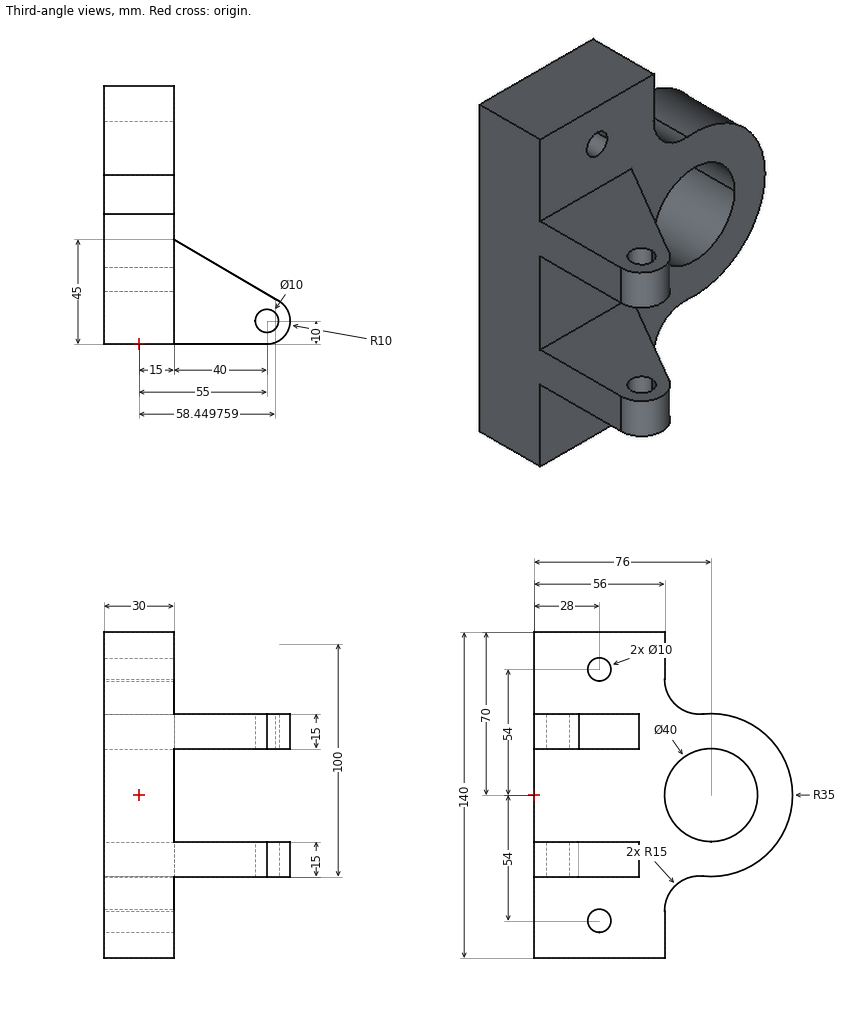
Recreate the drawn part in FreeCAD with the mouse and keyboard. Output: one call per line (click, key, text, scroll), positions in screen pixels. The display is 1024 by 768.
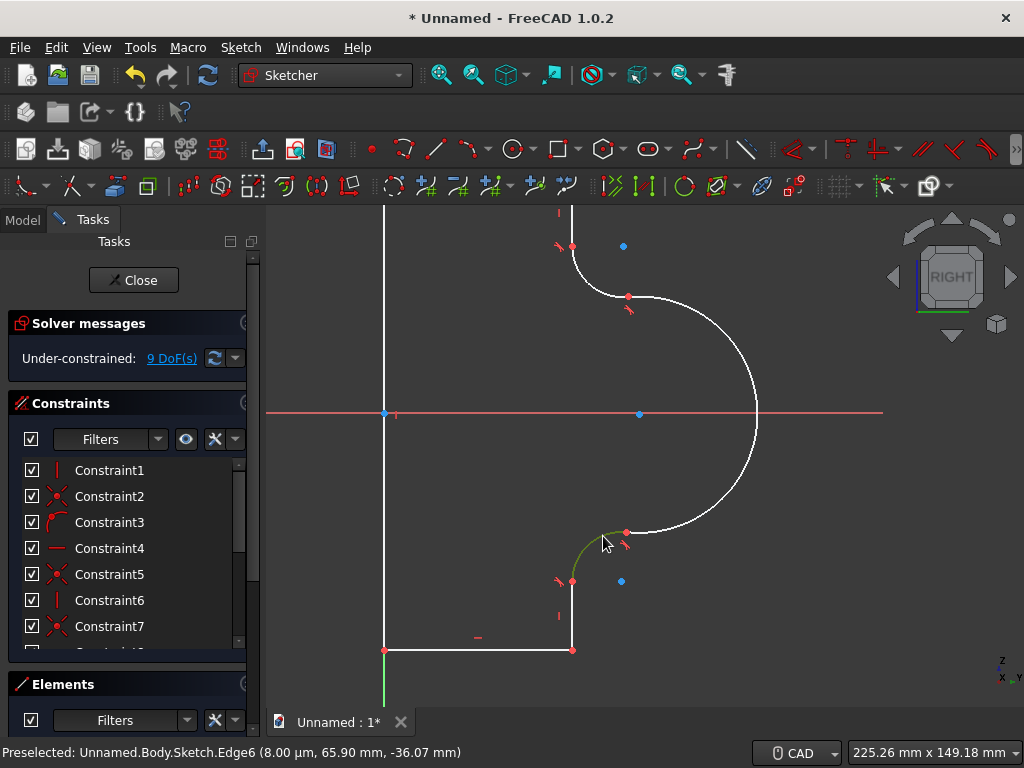
click(579, 271)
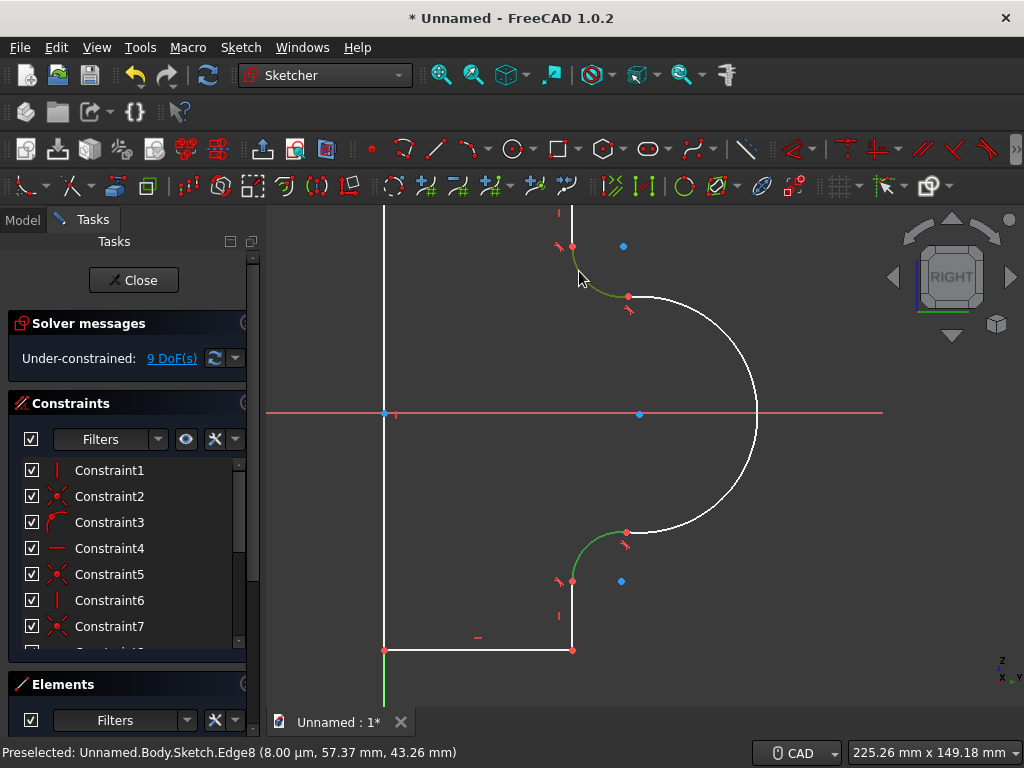
key(e)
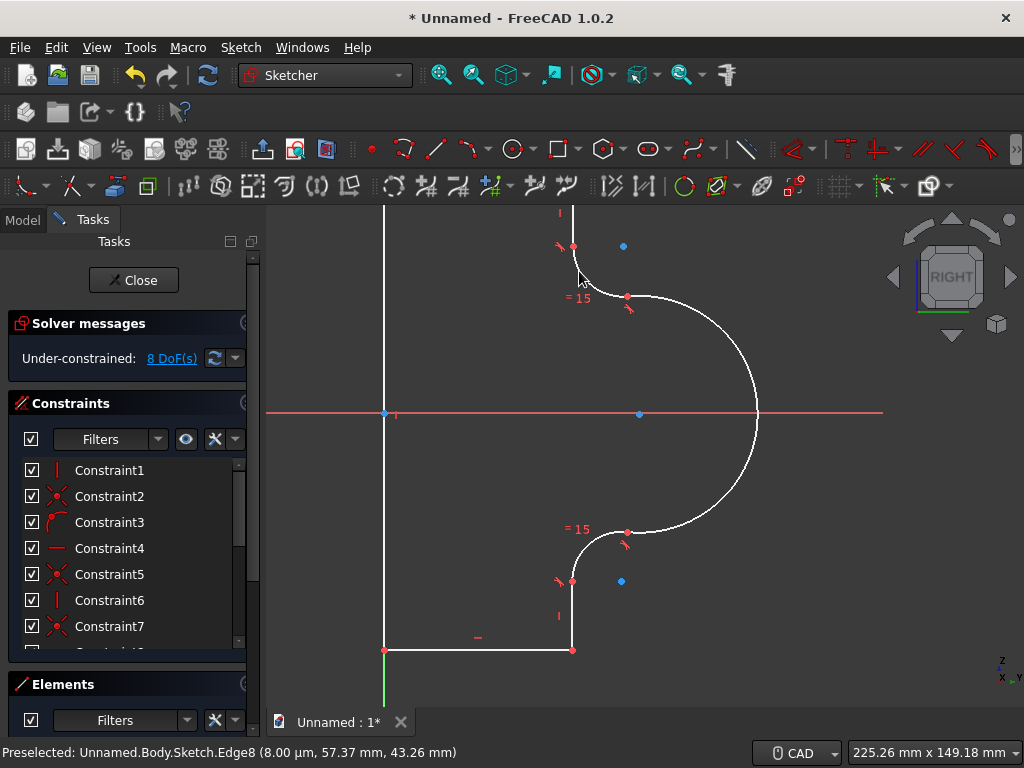
click(639, 414)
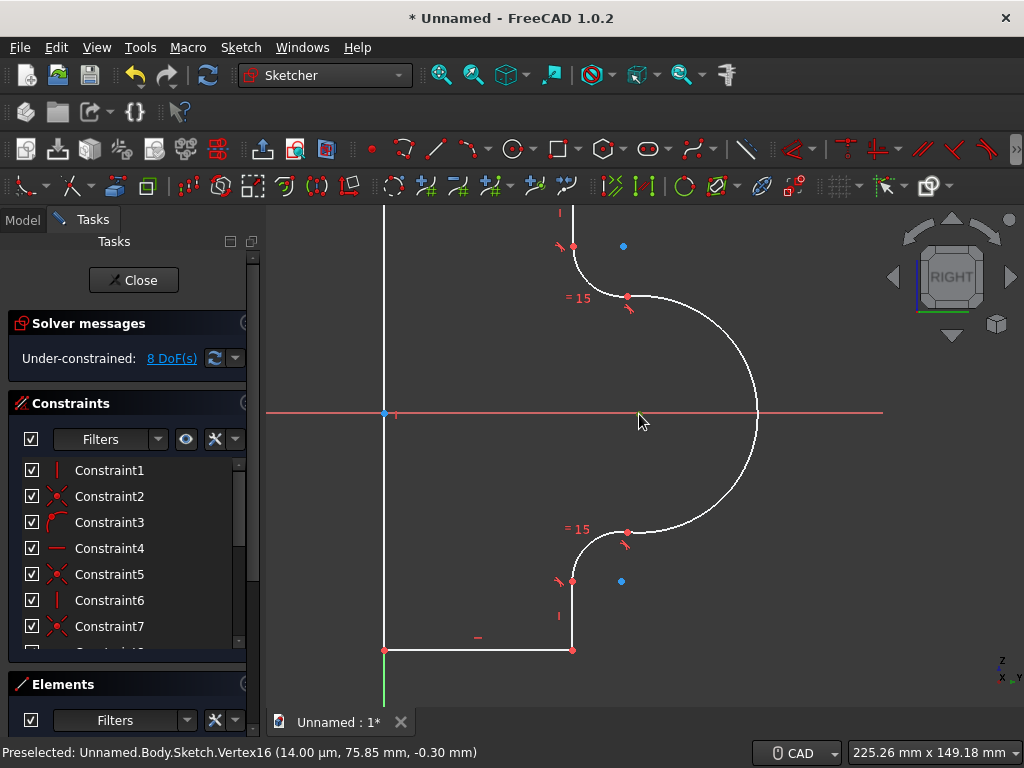
click(334, 413)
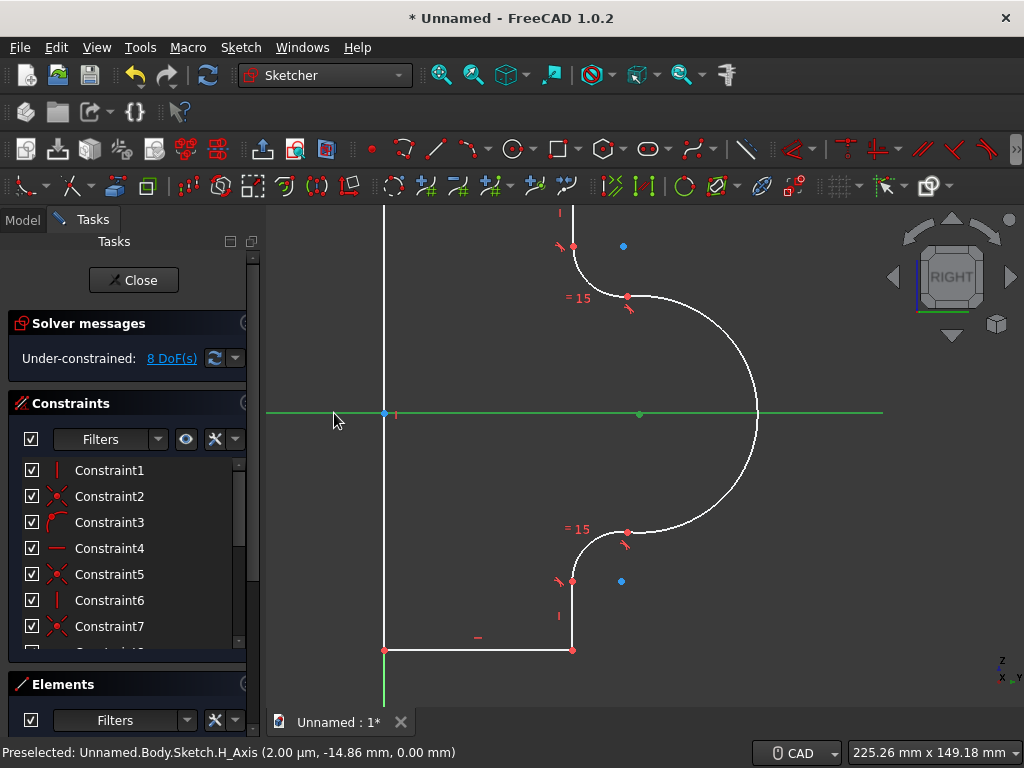
key(c)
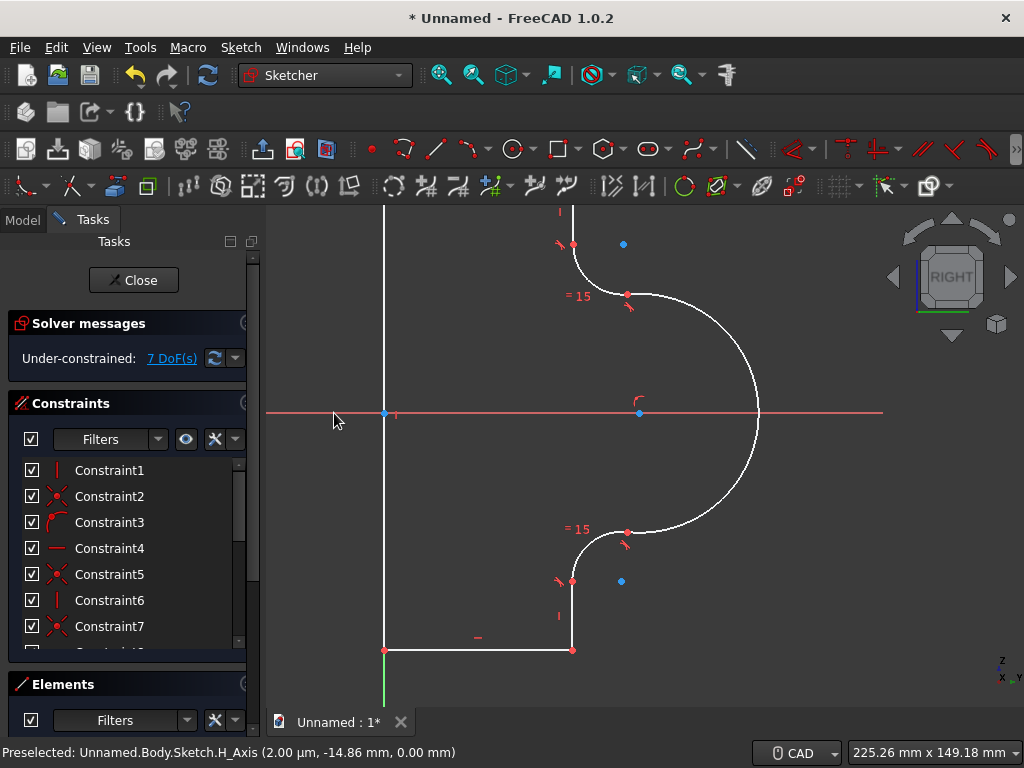
key(d)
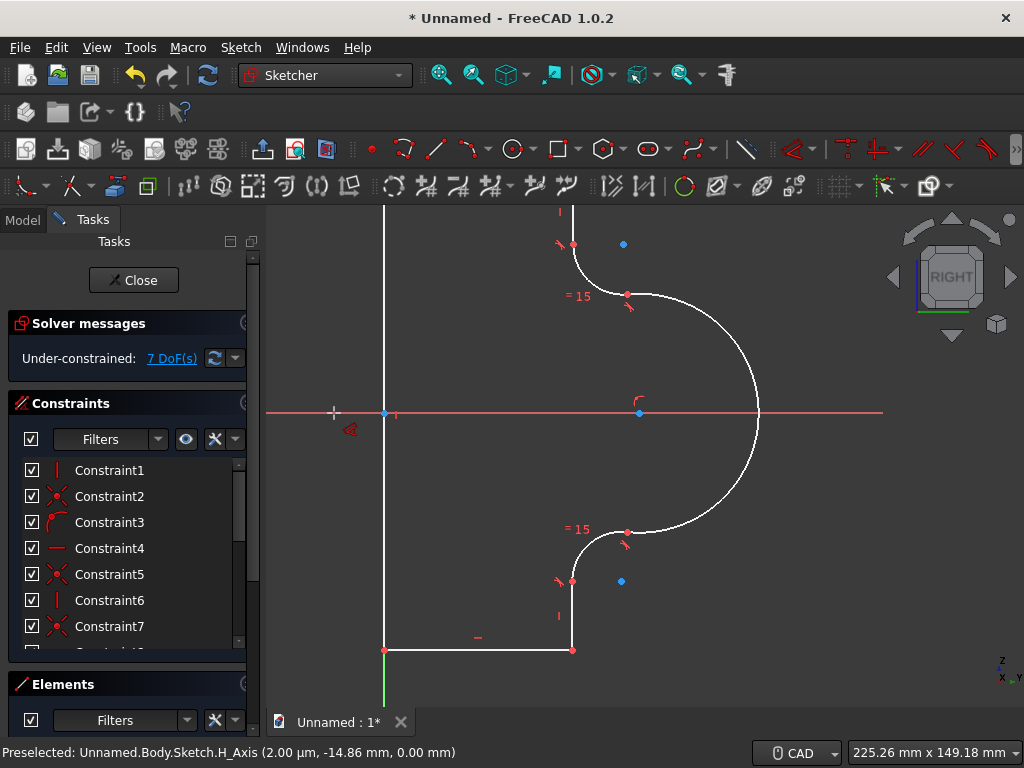
click(603, 536)
click(591, 506)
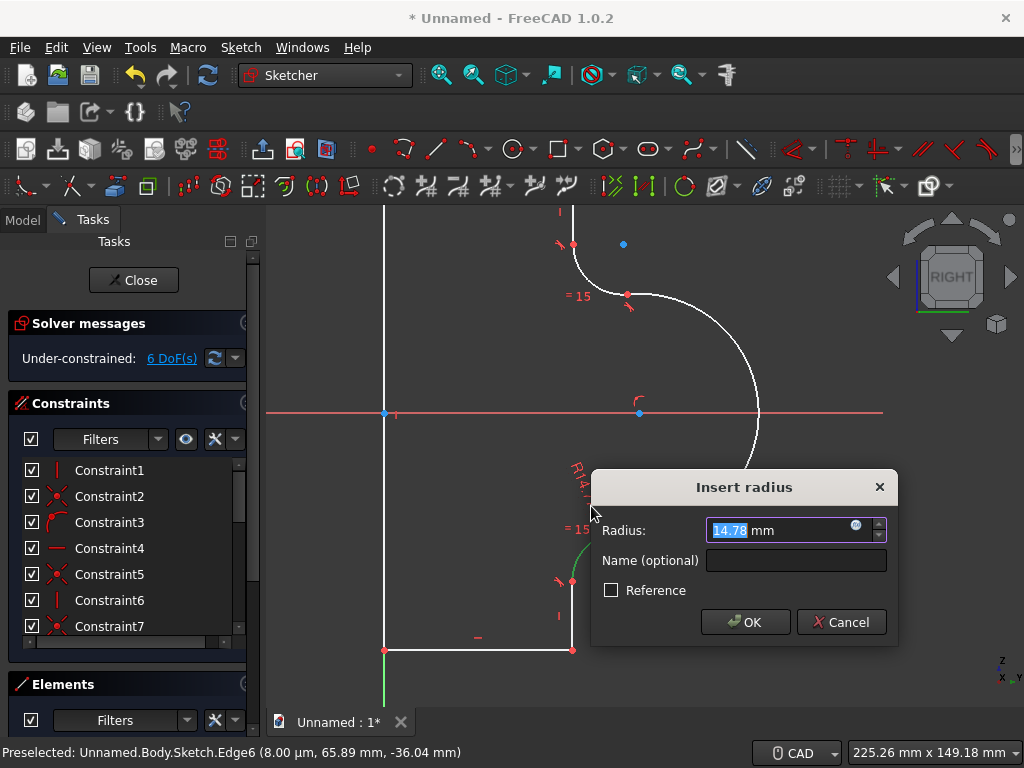
text(15)
key(Return)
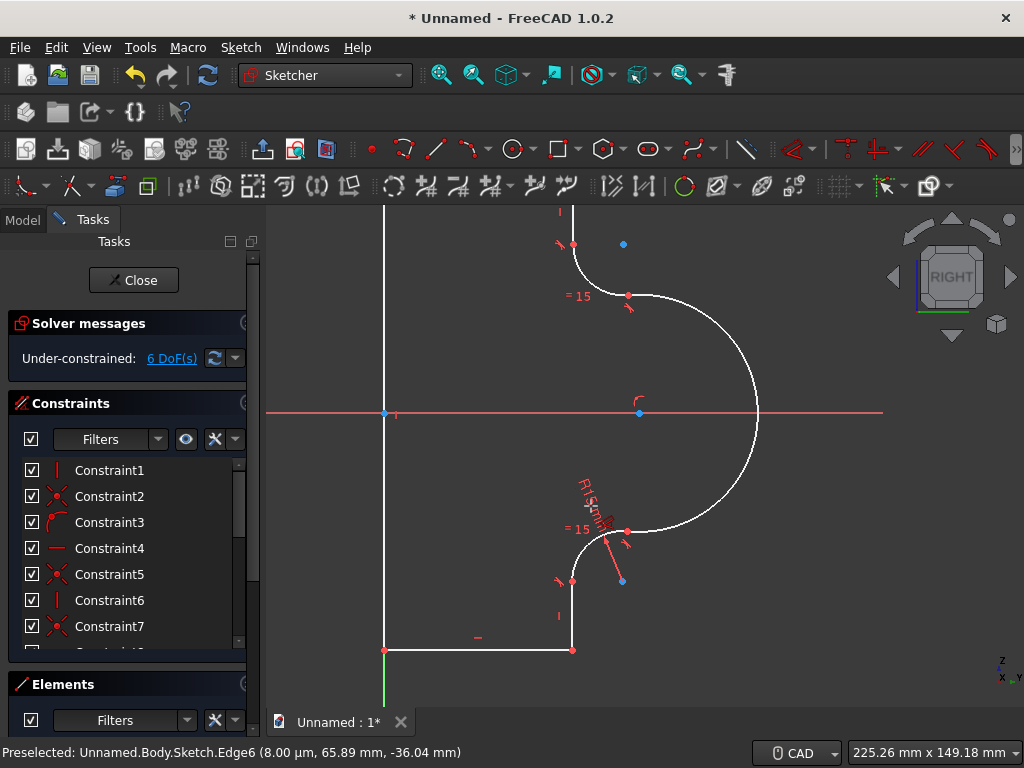
click(732, 487)
click(757, 507)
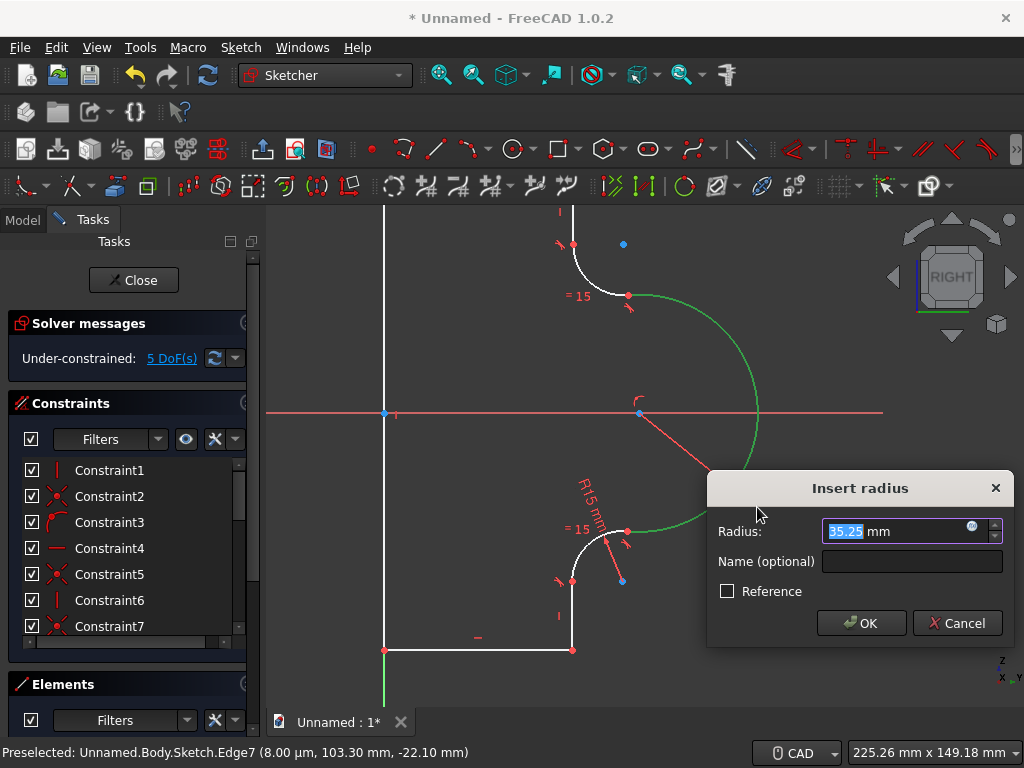
text(35)
key(Return)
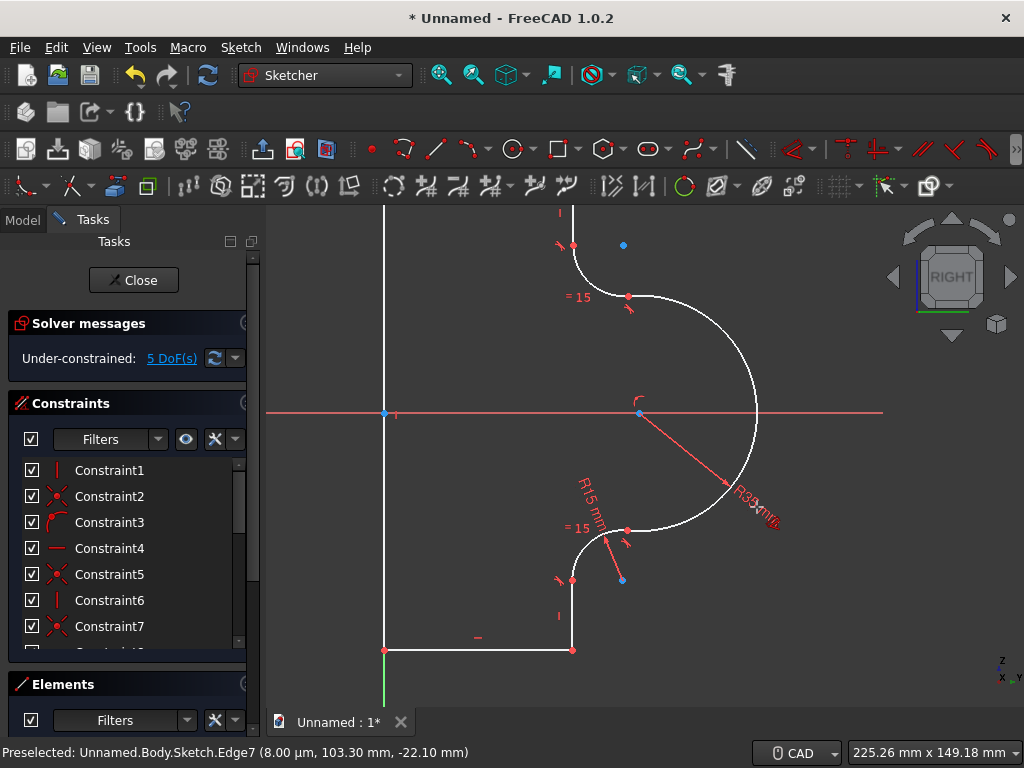
scroll(588, 543, down, 2)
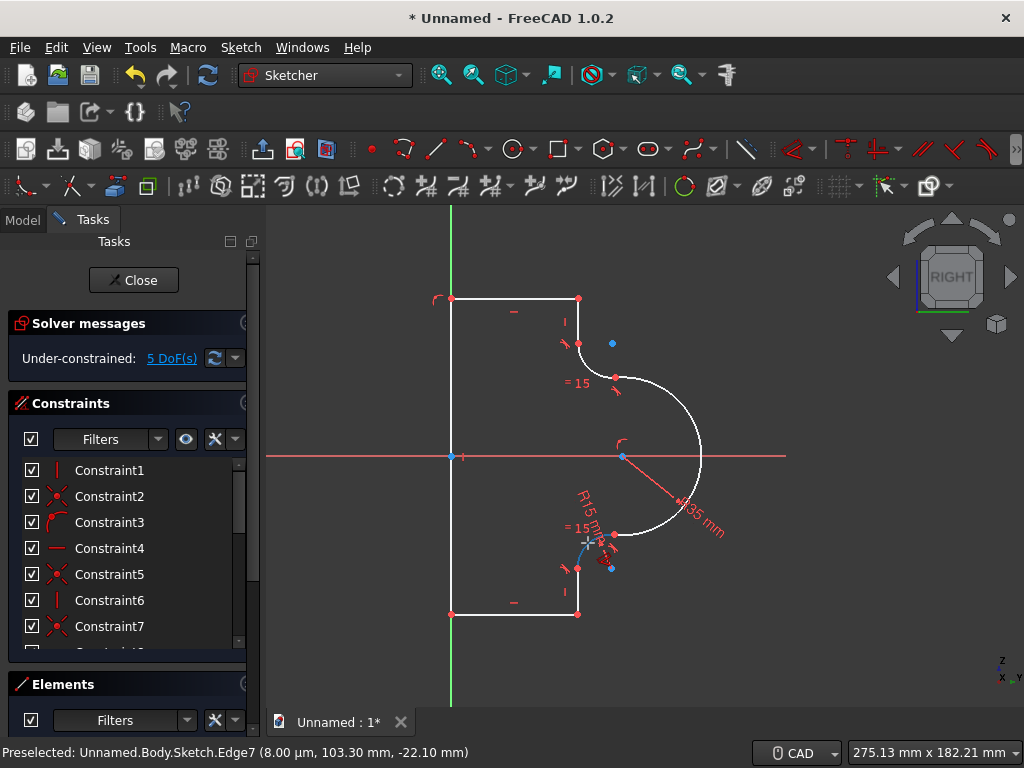
click(540, 299)
click(515, 265)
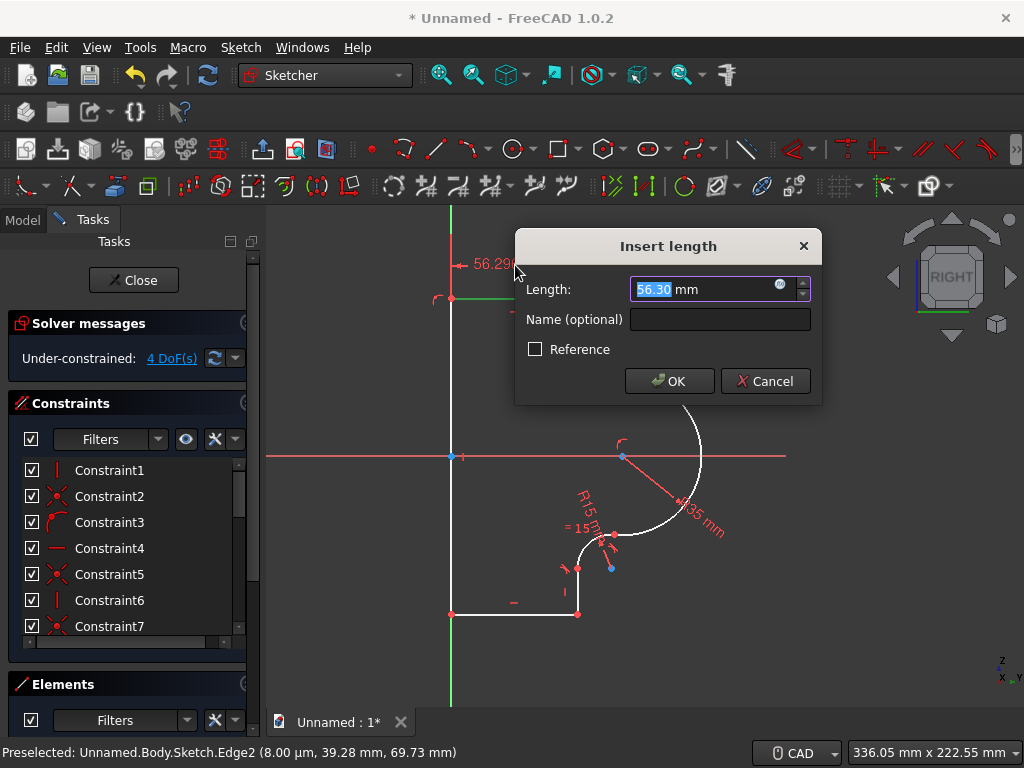
text(56)
key(Return)